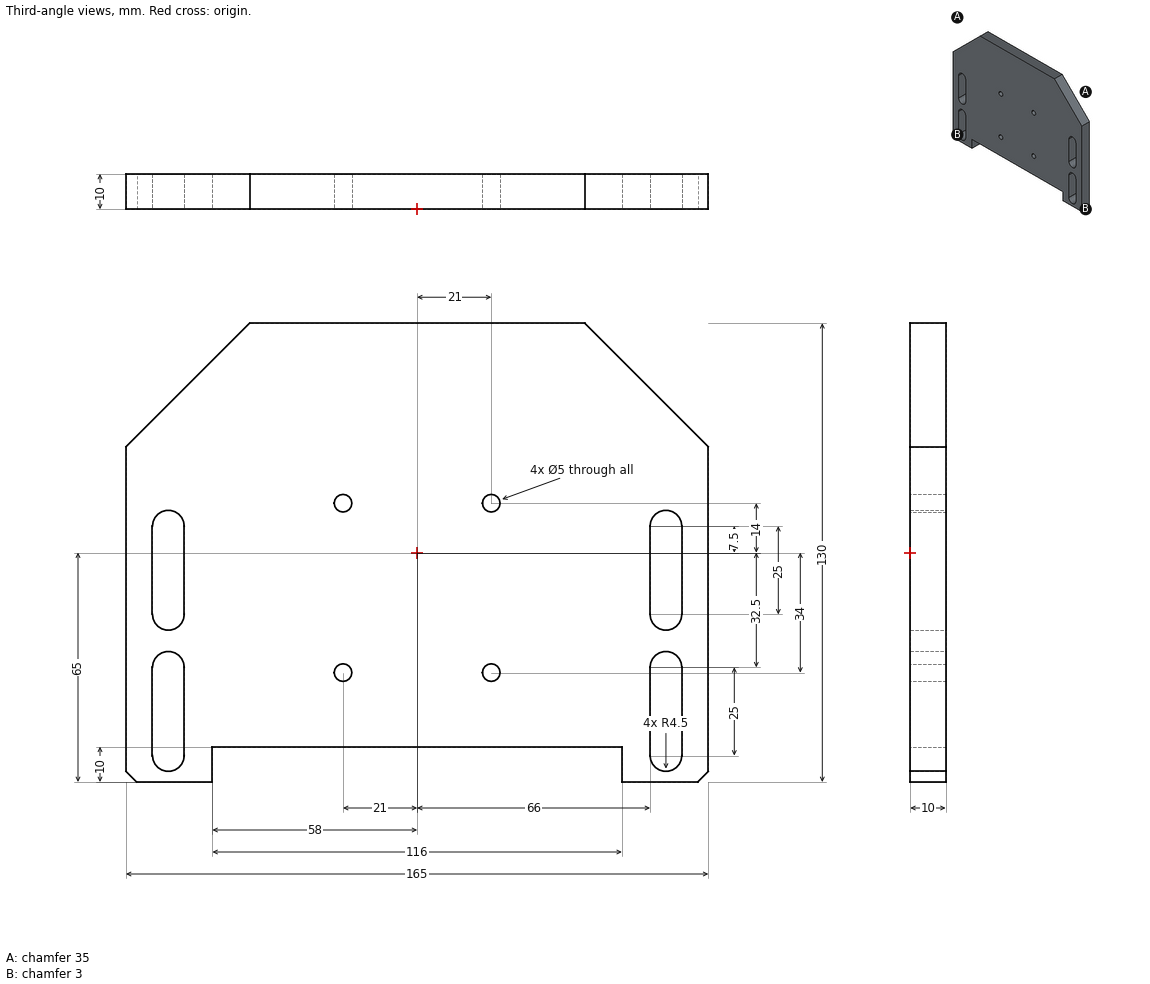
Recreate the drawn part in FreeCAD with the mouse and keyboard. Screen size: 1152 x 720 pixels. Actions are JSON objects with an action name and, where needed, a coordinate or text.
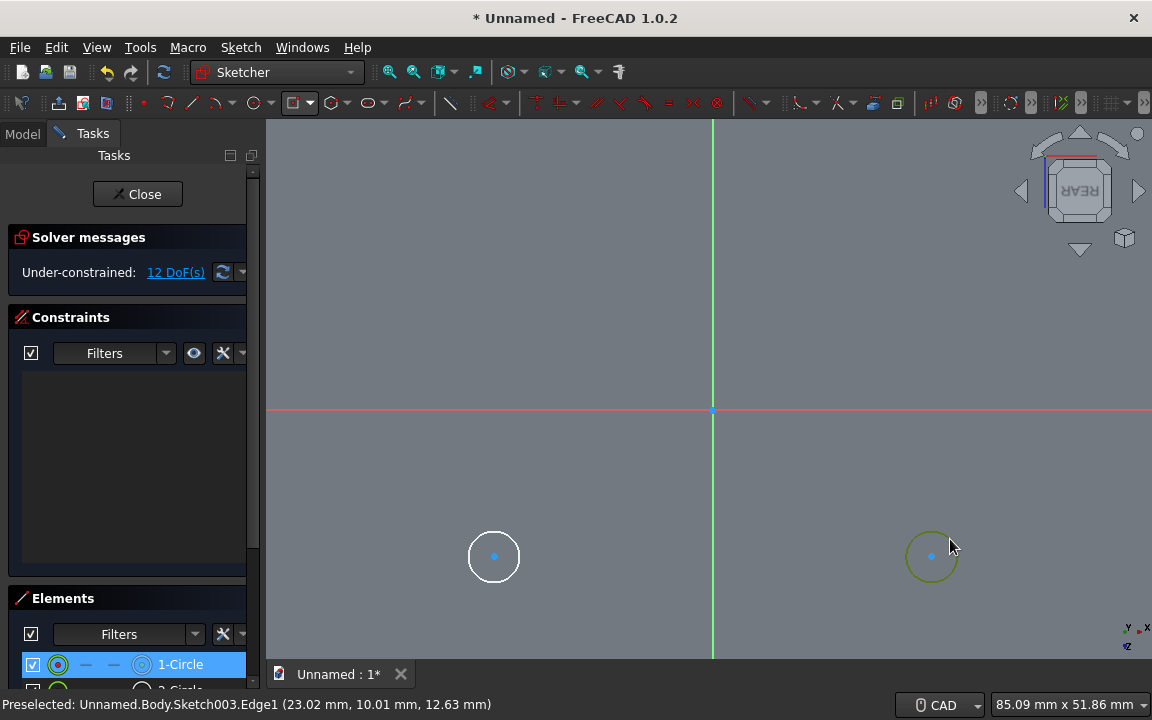
{"action": "scroll", "coordinate": [494, 557], "scroll_direction": "down", "scroll_amount": 2}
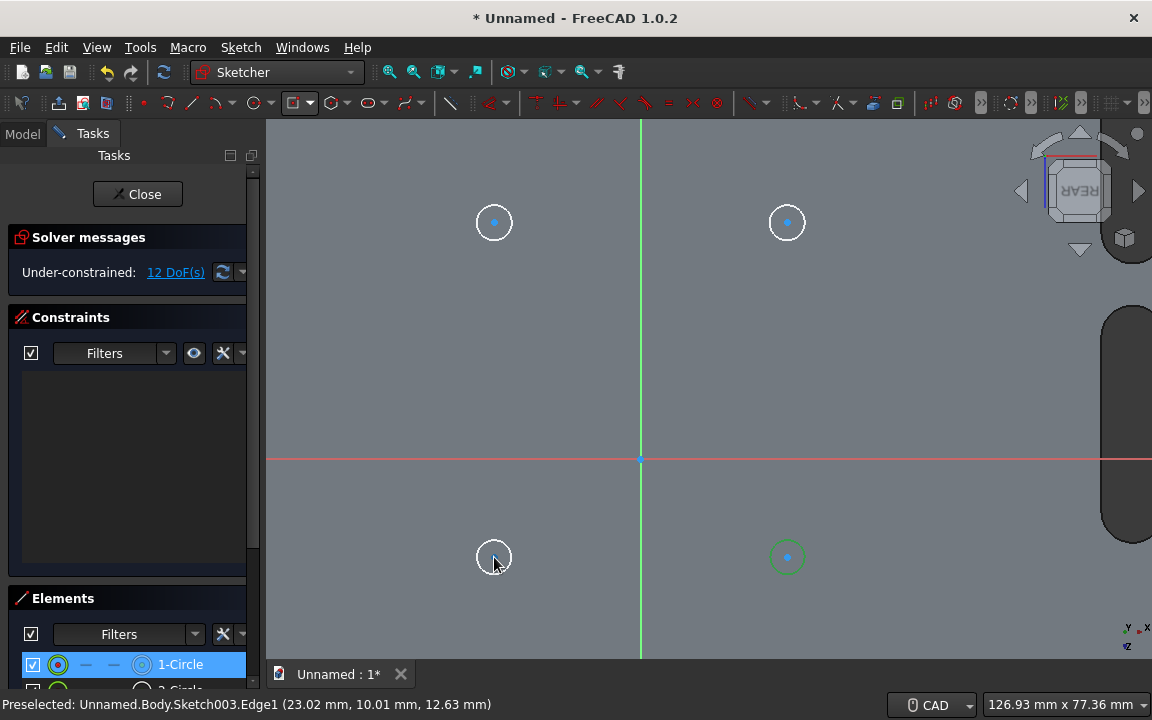
{"action": "left_click", "coordinate": [800, 210]}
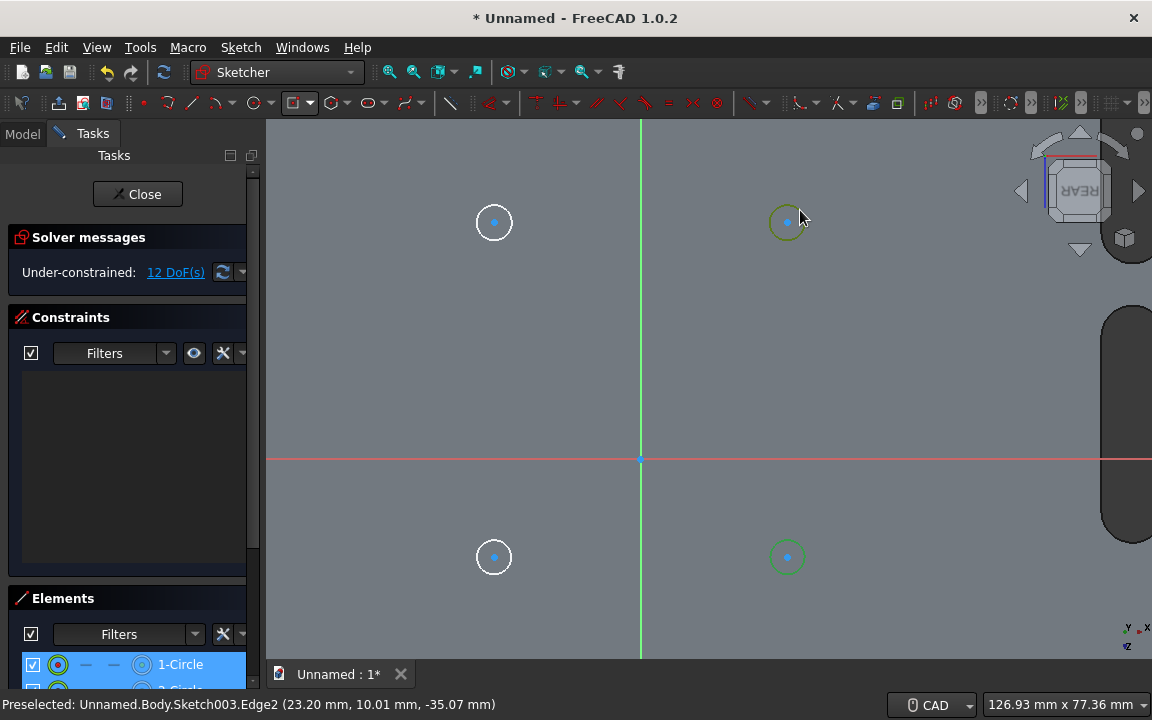
{"action": "left_click", "coordinate": [507, 210]}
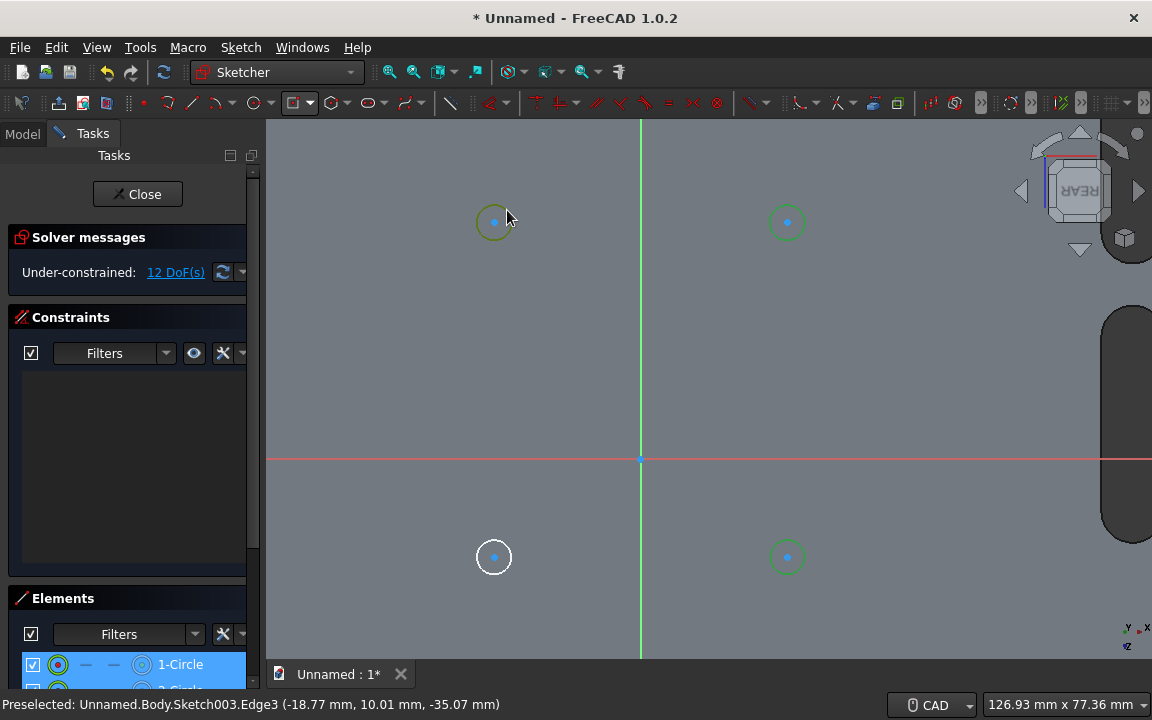
{"action": "left_click", "coordinate": [506, 545]}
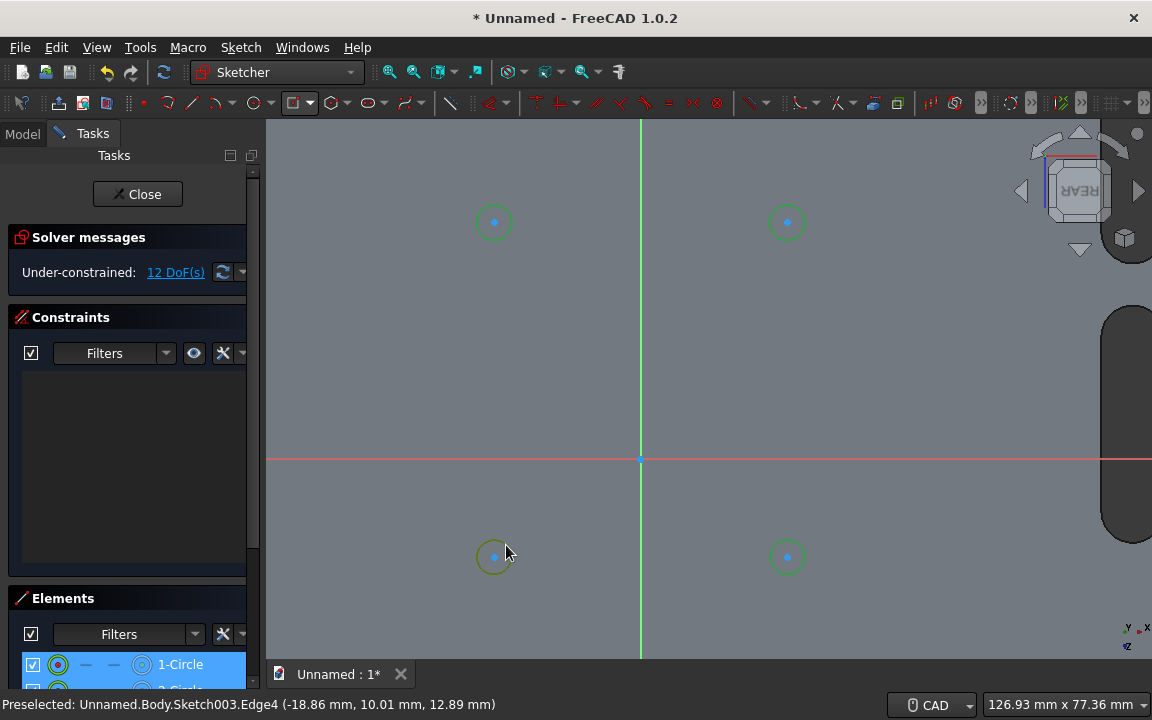
{"action": "key", "text": "e"}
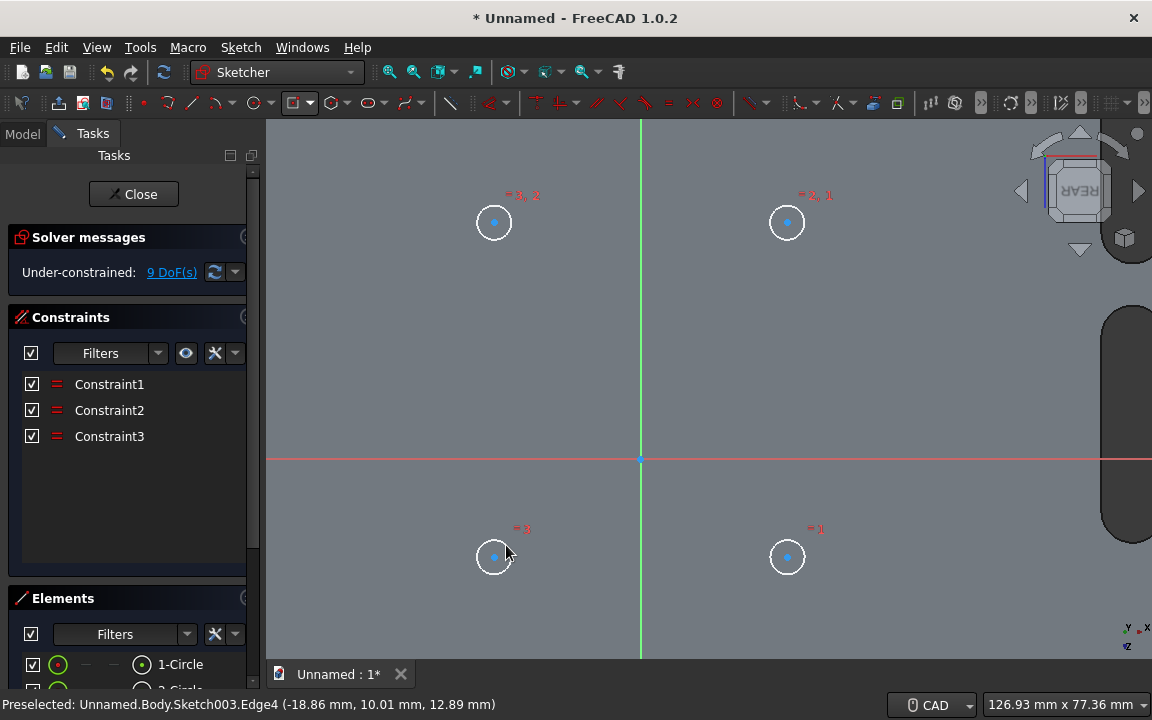
{"action": "left_click", "coordinate": [788, 557]}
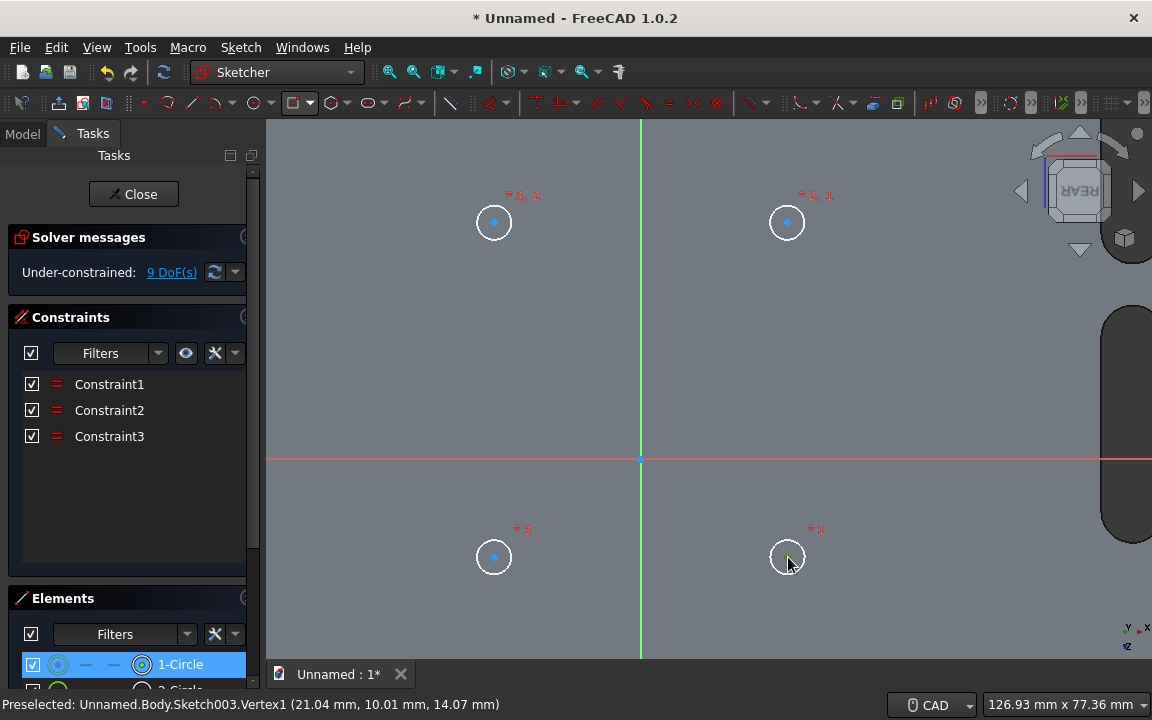
{"action": "left_click", "coordinate": [787, 223]}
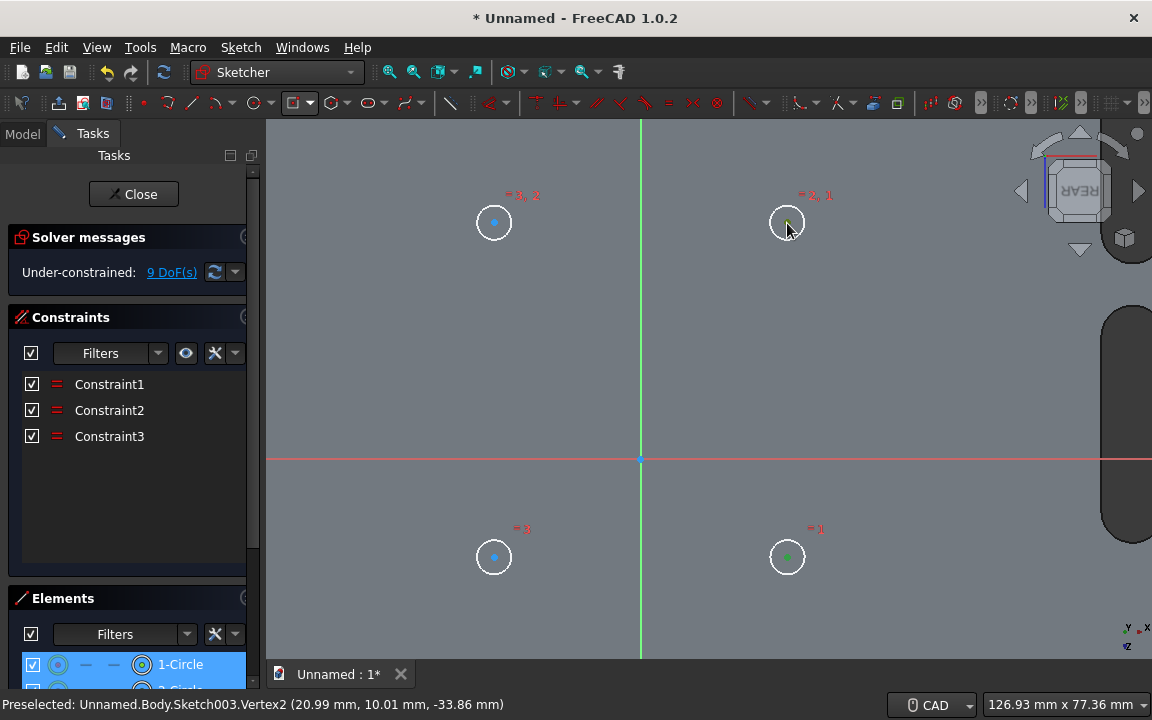
{"action": "key", "text": "v"}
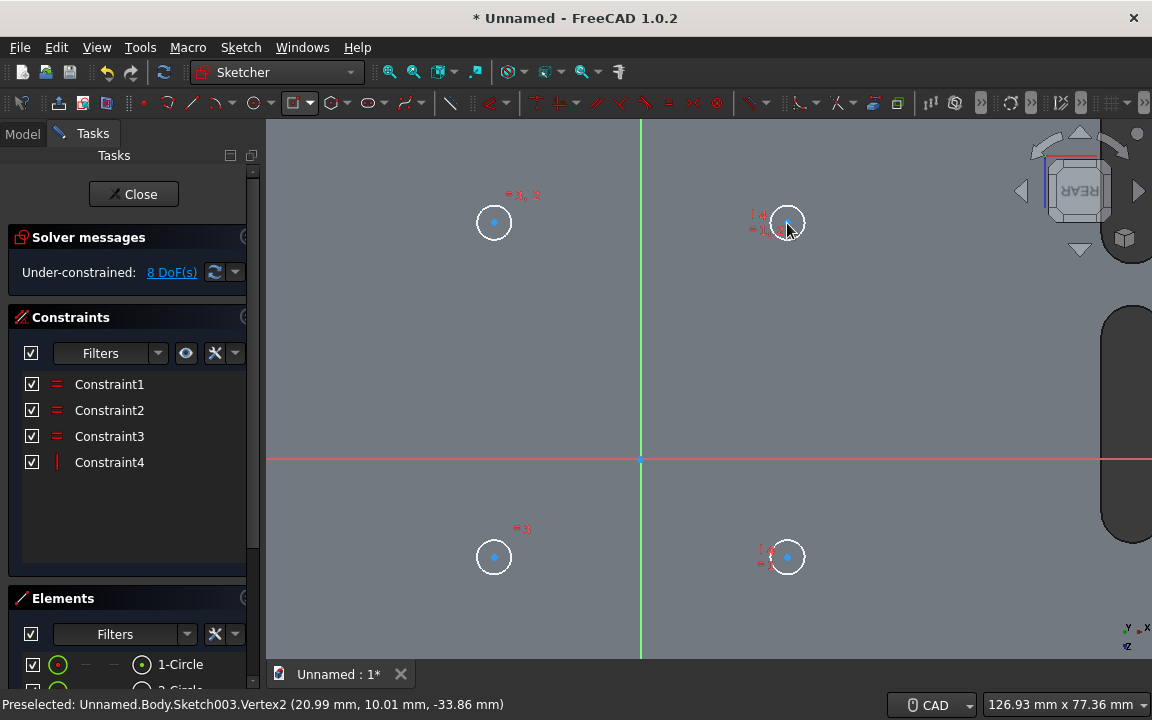
{"action": "left_click", "coordinate": [788, 223]}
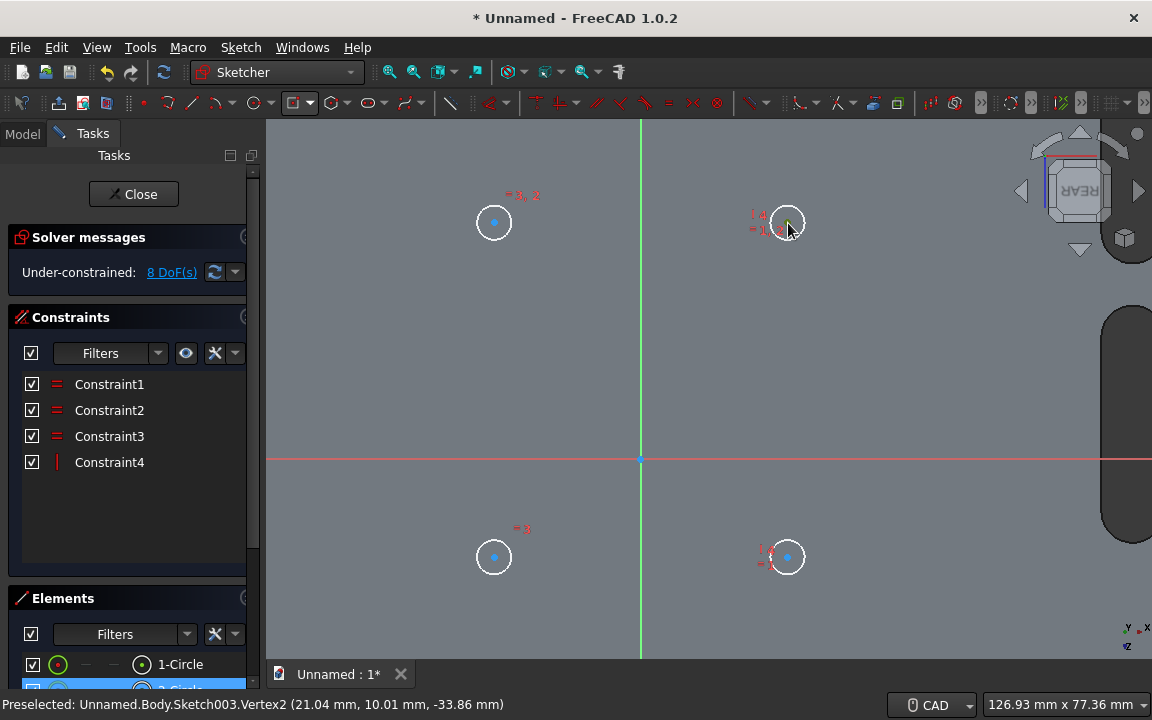
{"action": "left_click", "coordinate": [494, 223]}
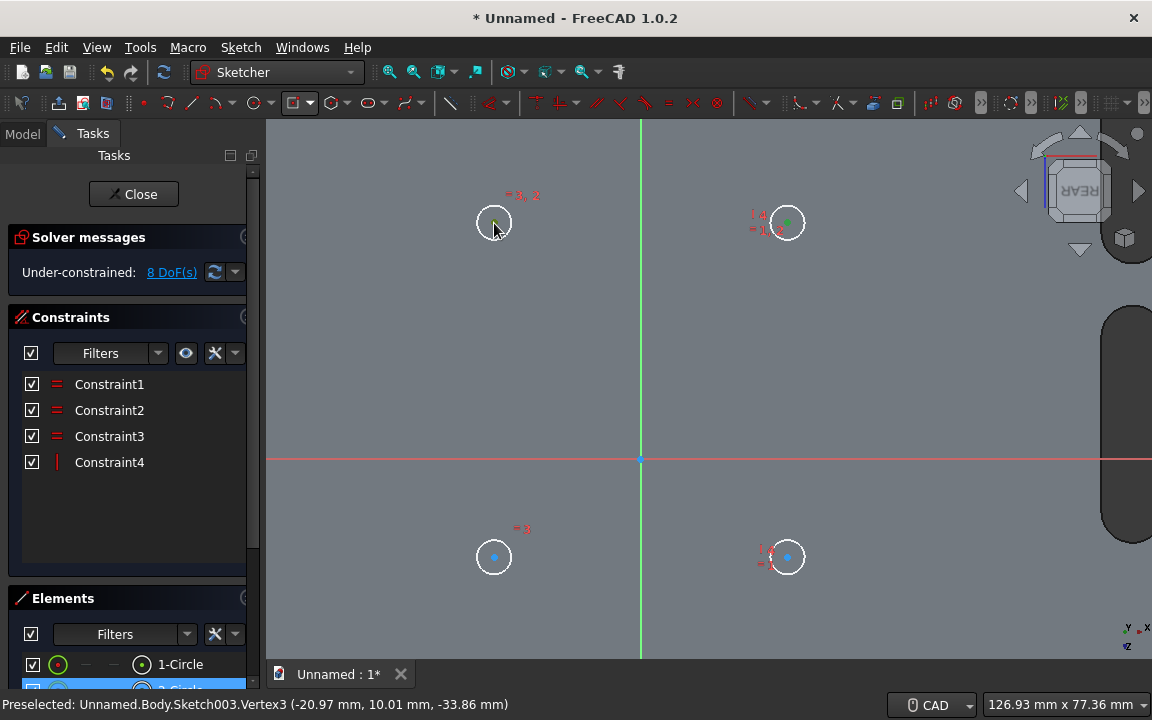
{"action": "key", "text": "h"}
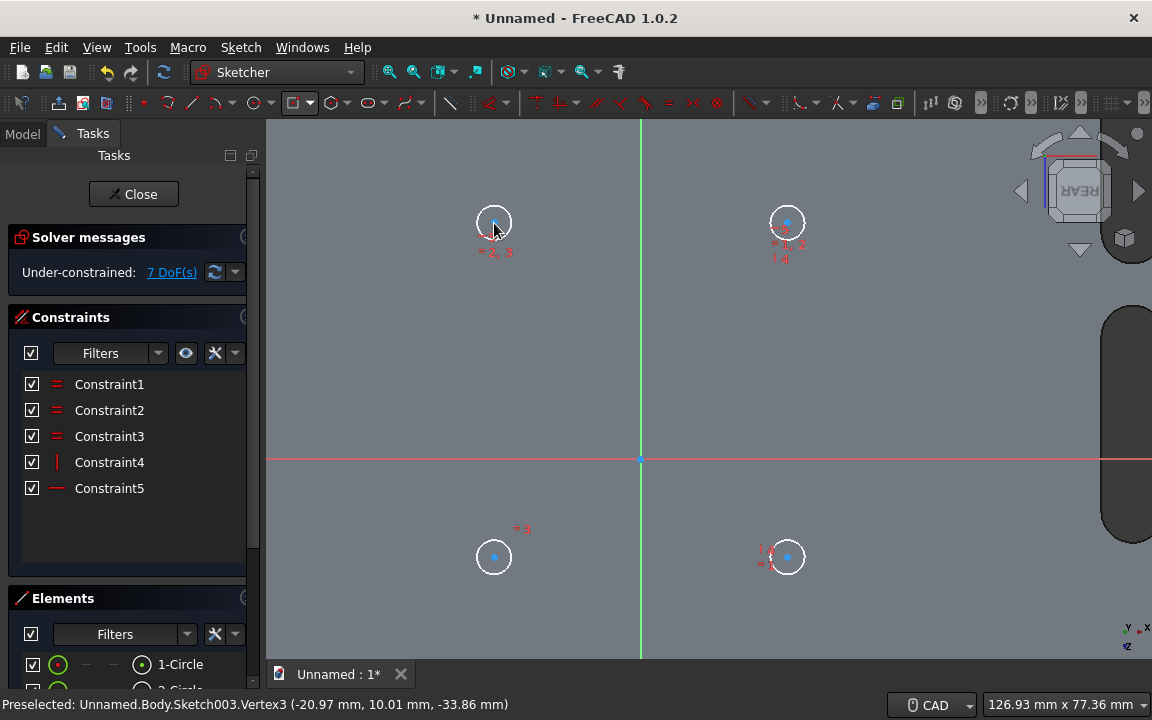
{"action": "left_click", "coordinate": [494, 223]}